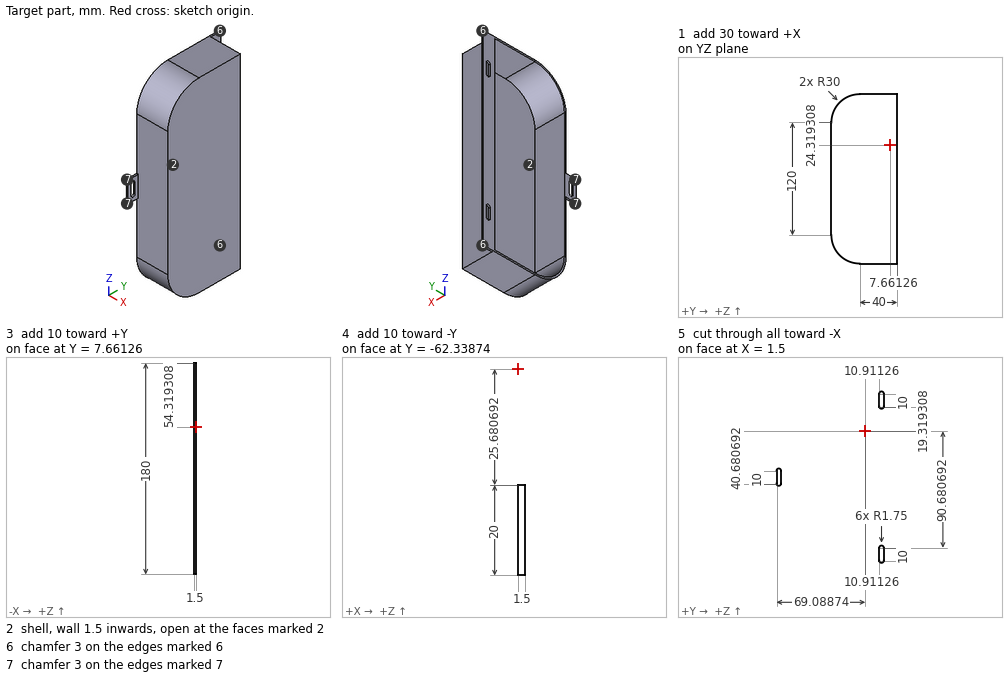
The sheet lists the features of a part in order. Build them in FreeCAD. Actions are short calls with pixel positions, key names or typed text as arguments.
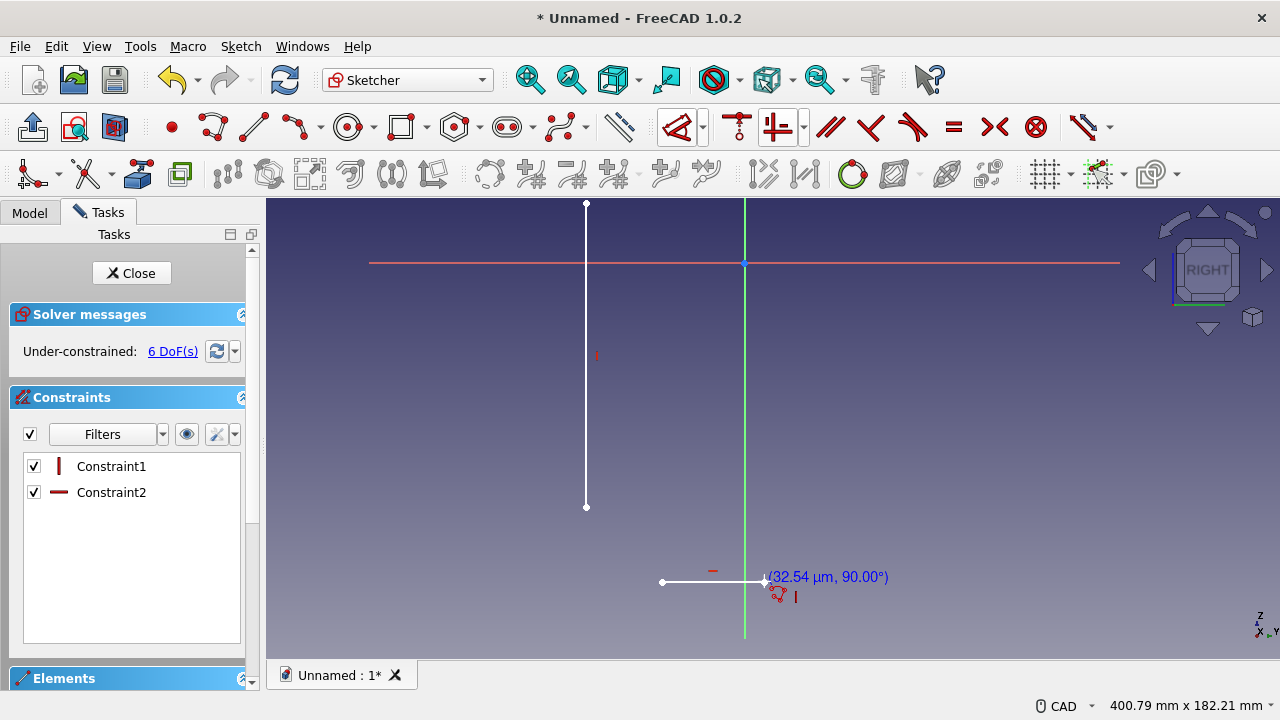
scroll(764, 581, down, 2)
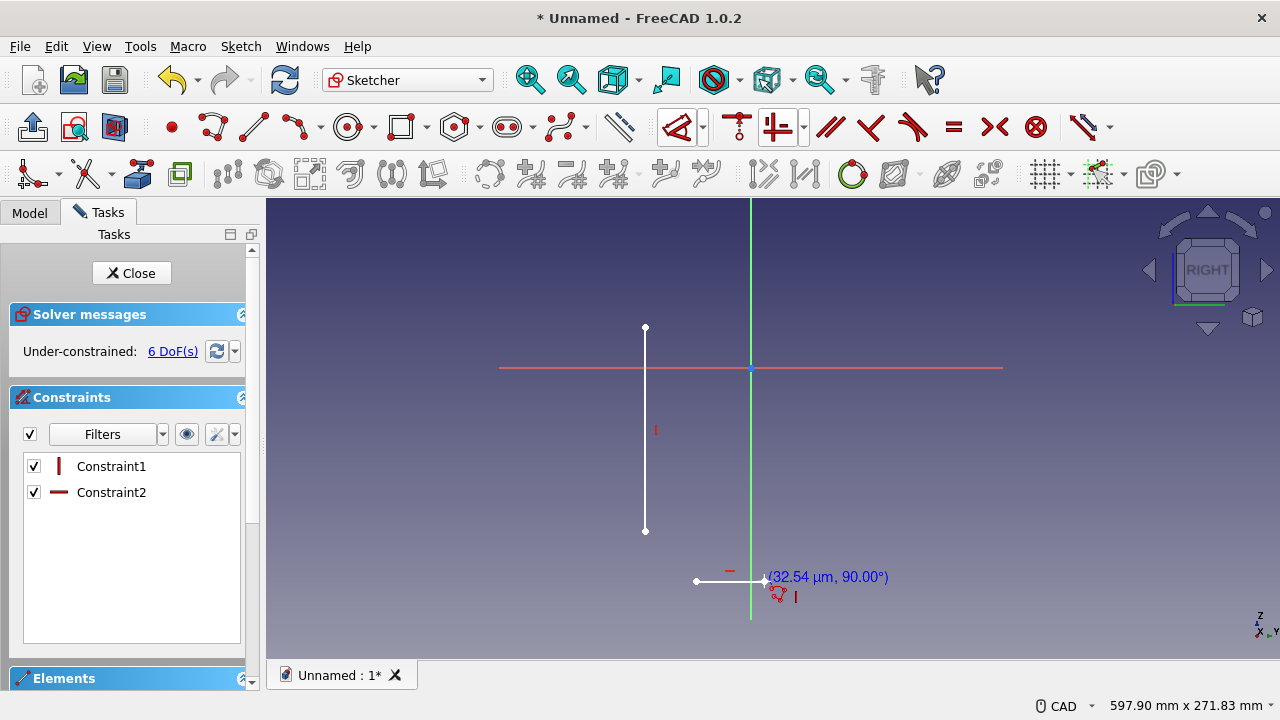
scroll(764, 276, up, 2)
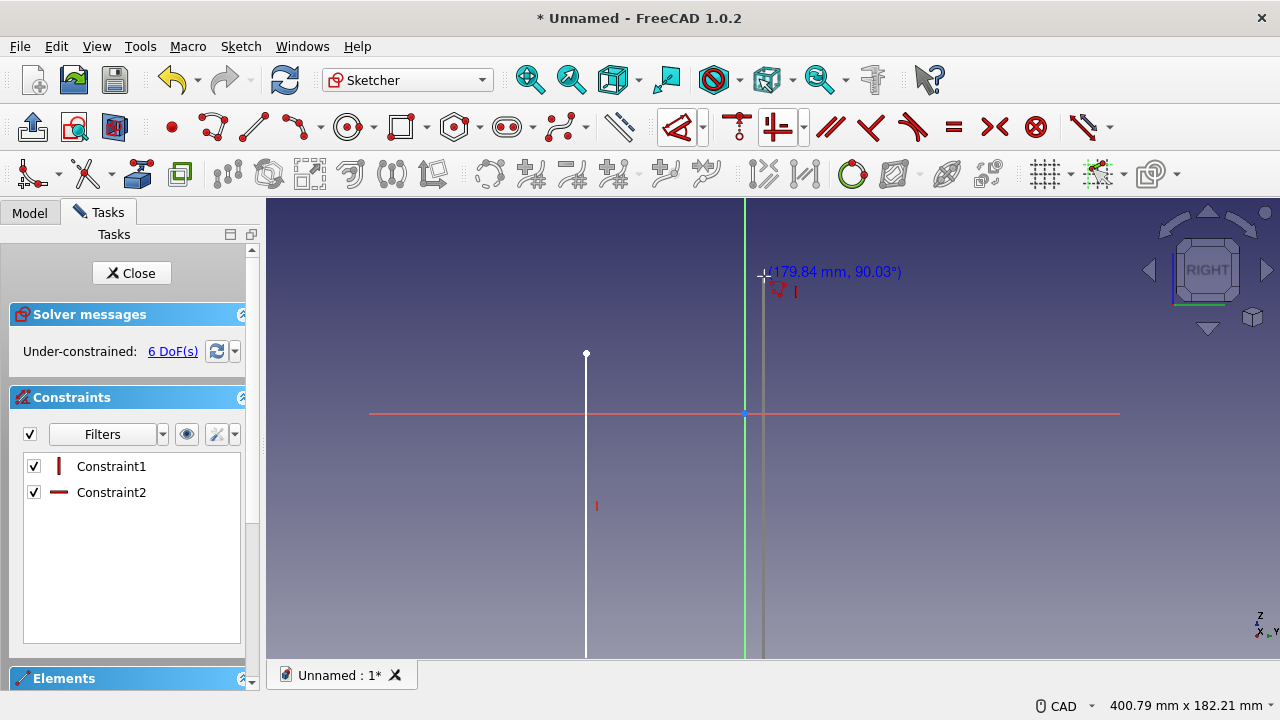
click(764, 276)
click(663, 276)
right_click(663, 276)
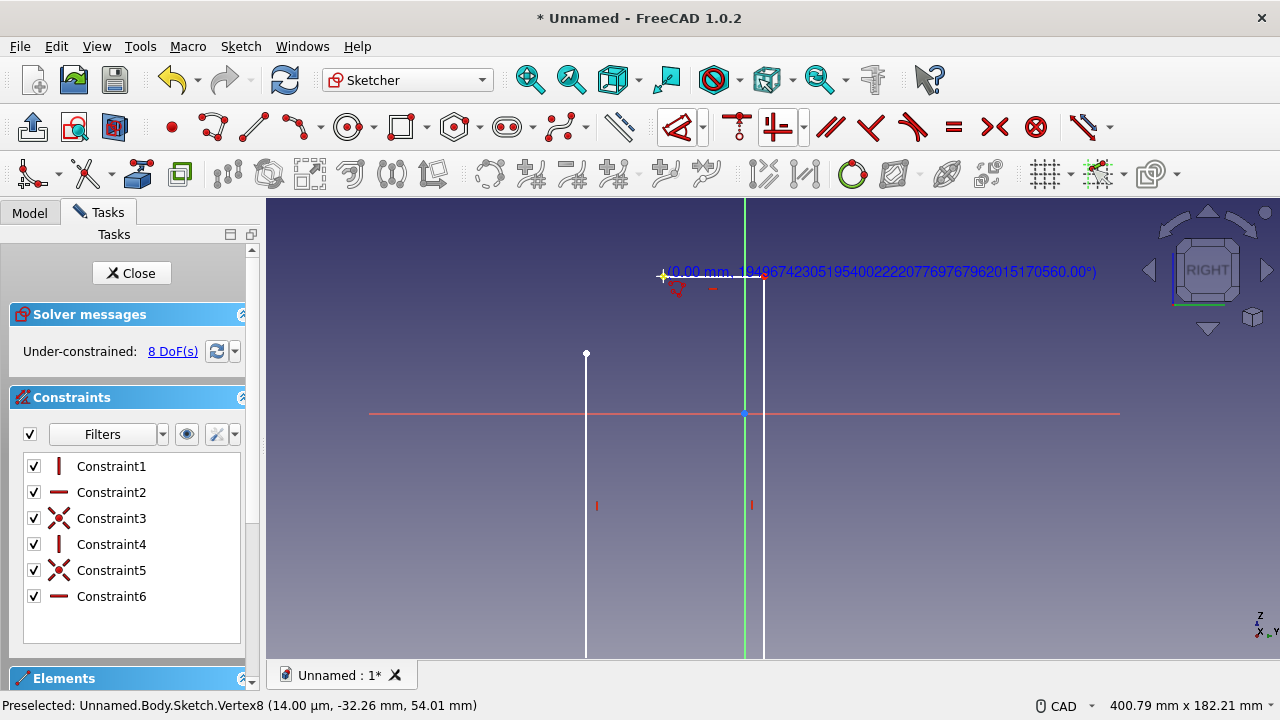
click(294, 128)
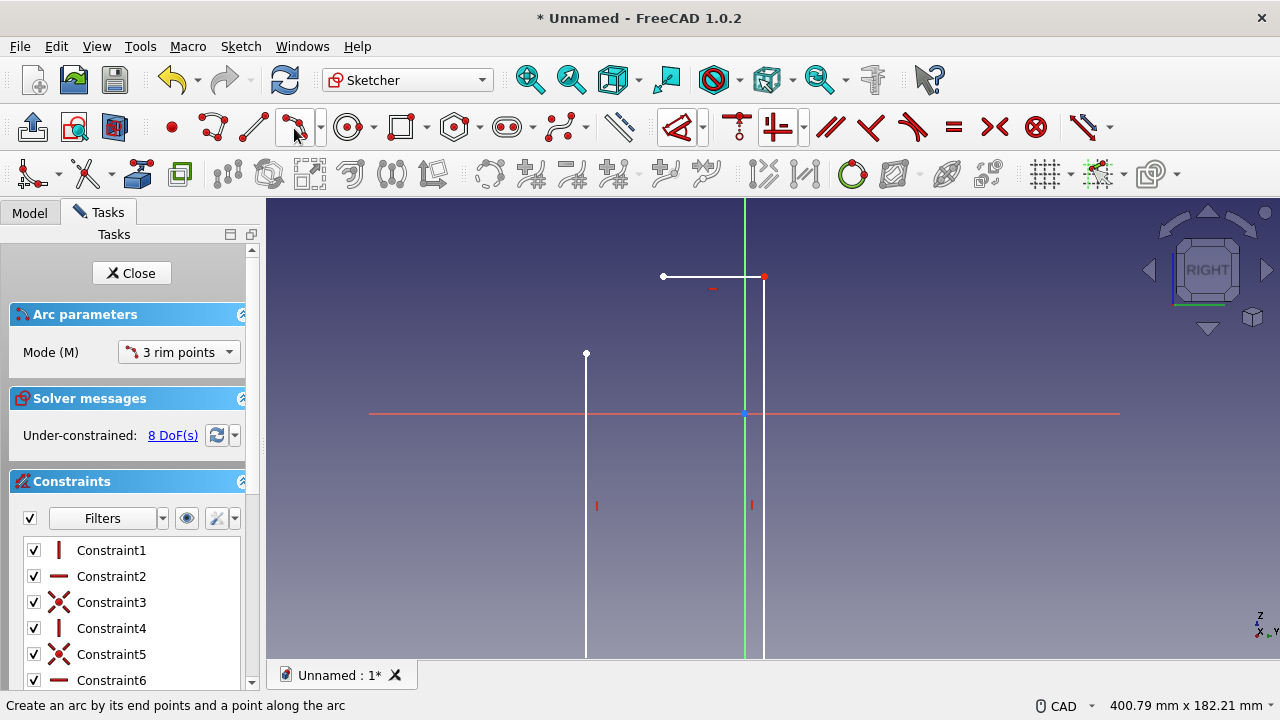
scroll(764, 275, down, 2)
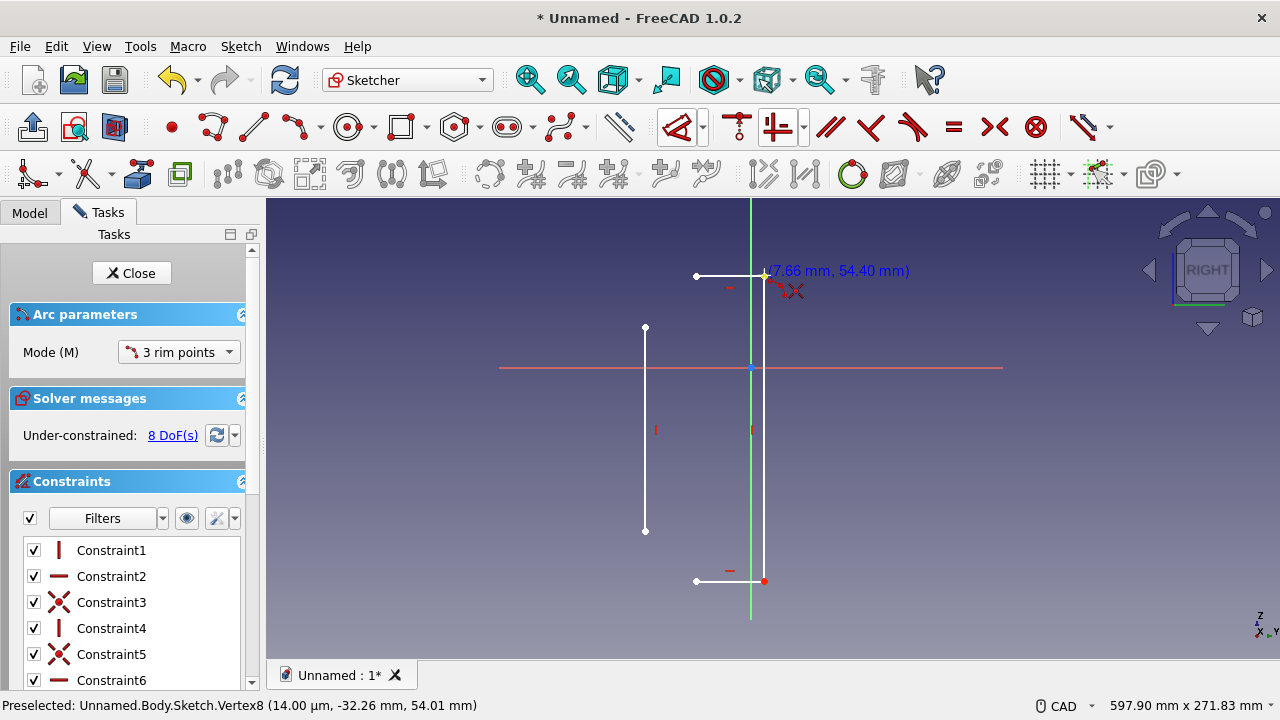
click(645, 532)
click(696, 582)
click(660, 566)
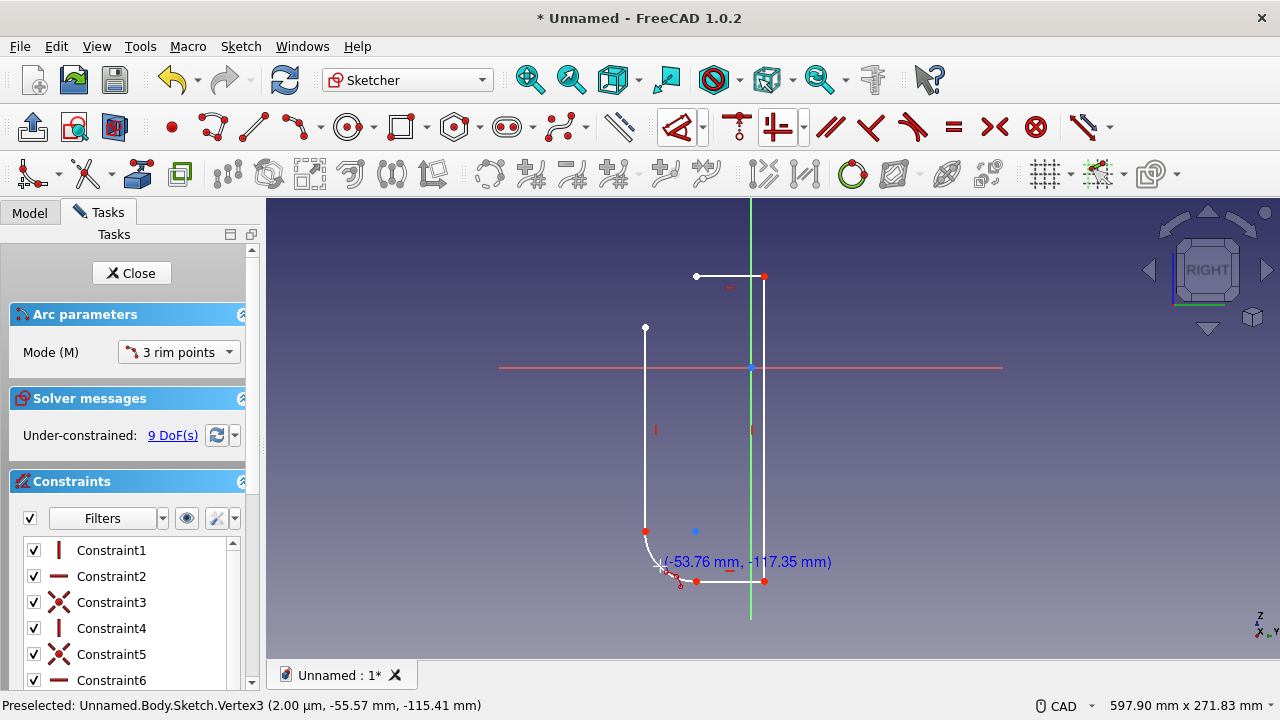
click(696, 276)
click(645, 328)
click(660, 291)
key(Escape)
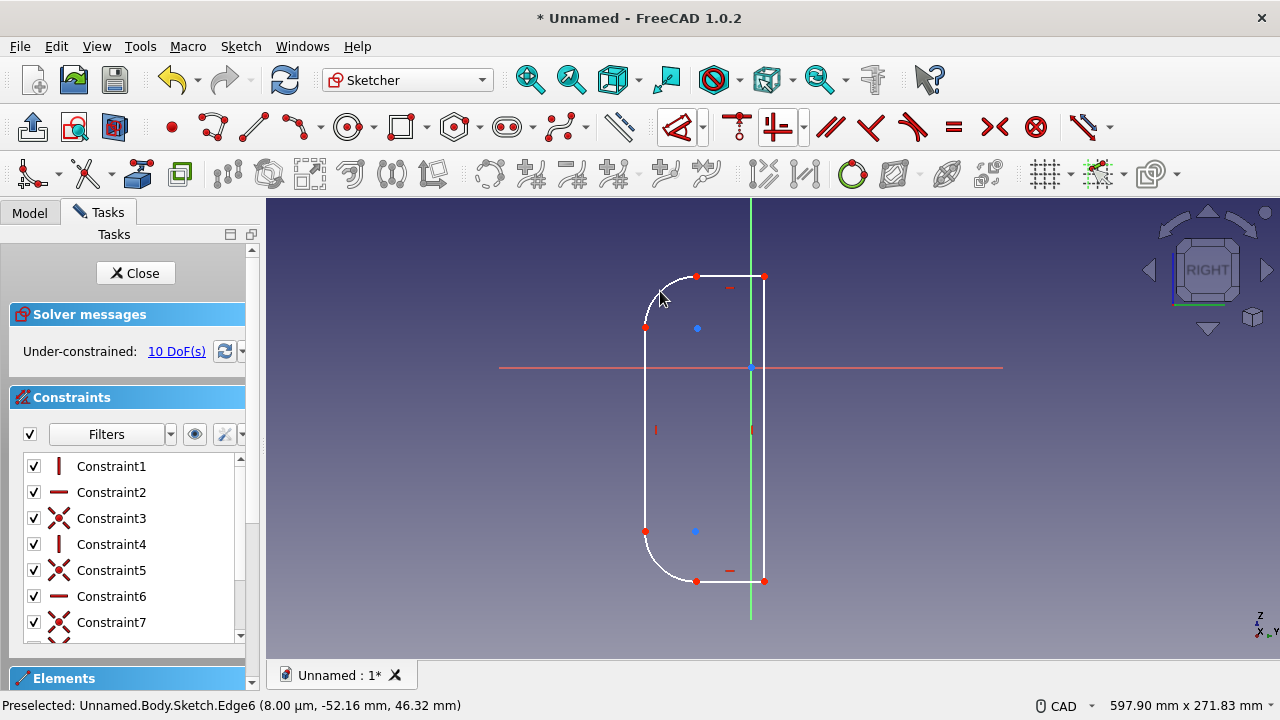
click(645, 389)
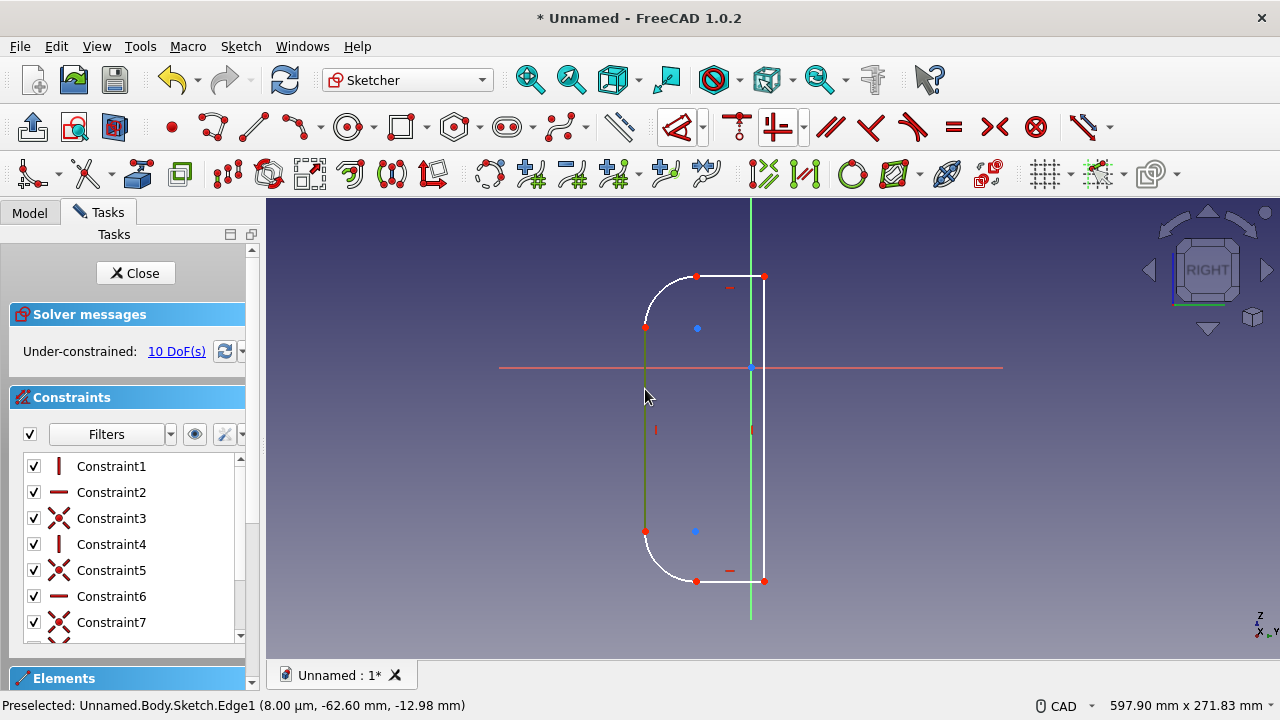
click(651, 555)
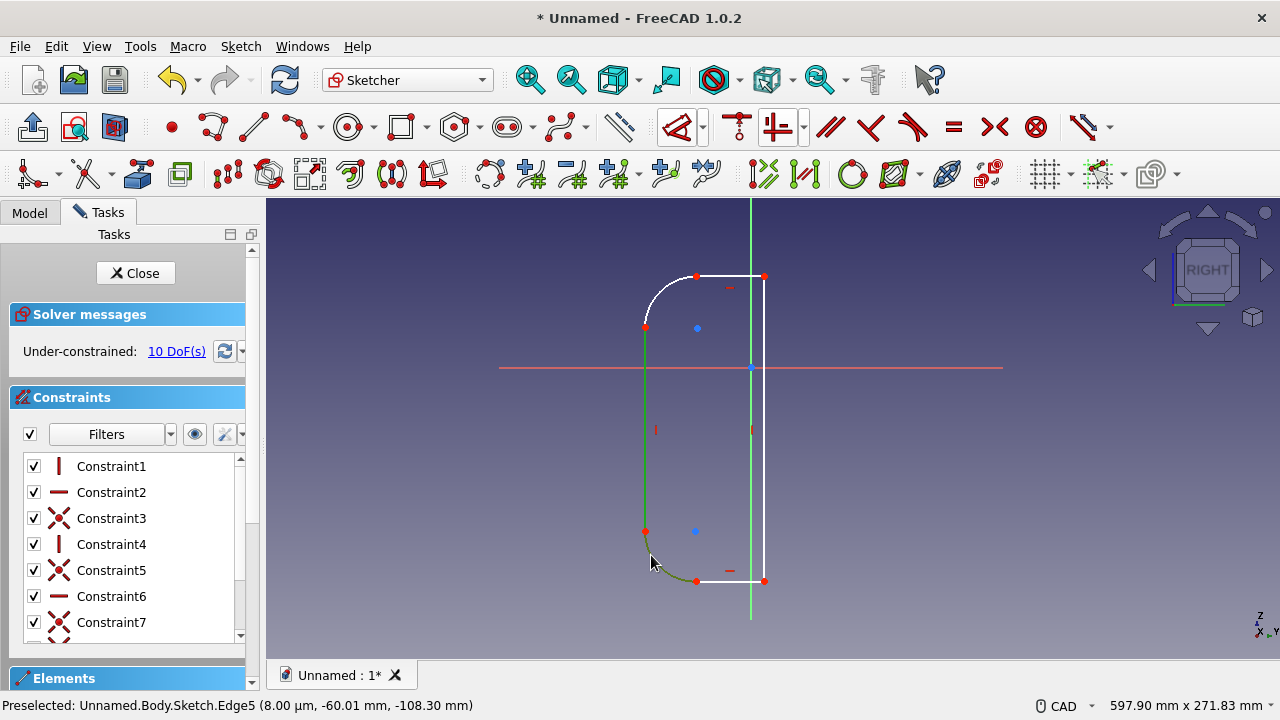
click(913, 128)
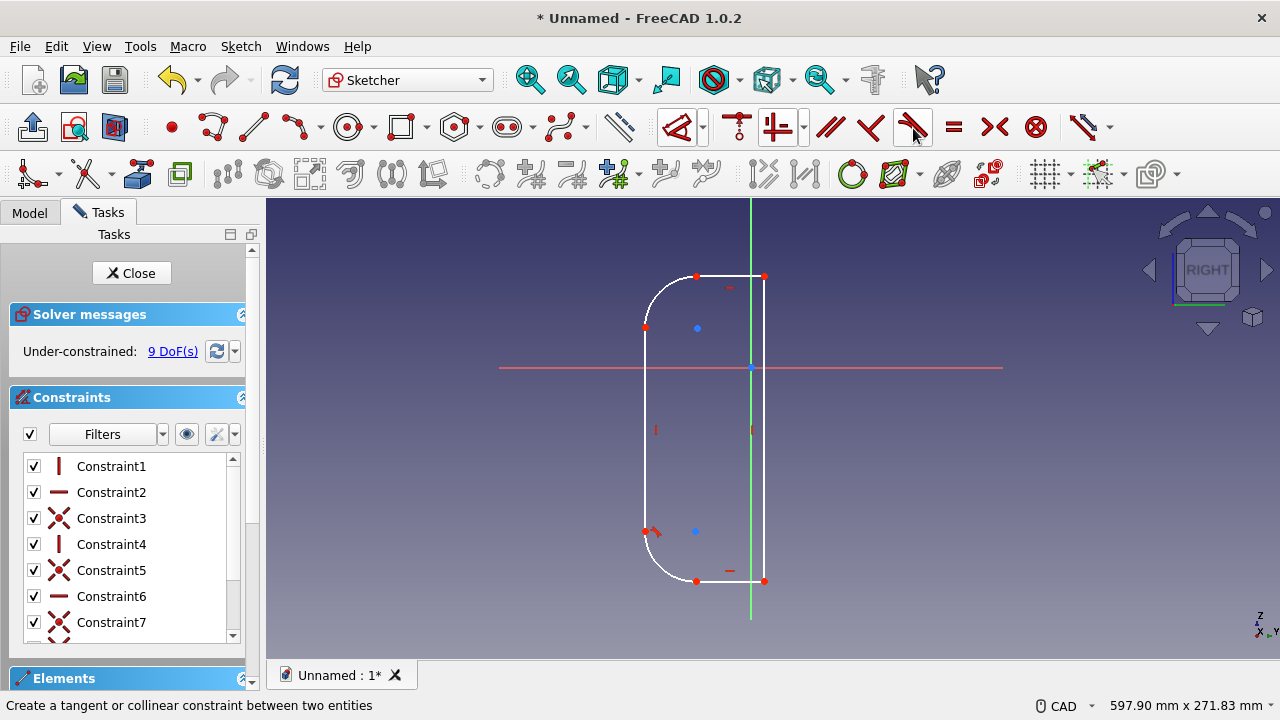
click(645, 389)